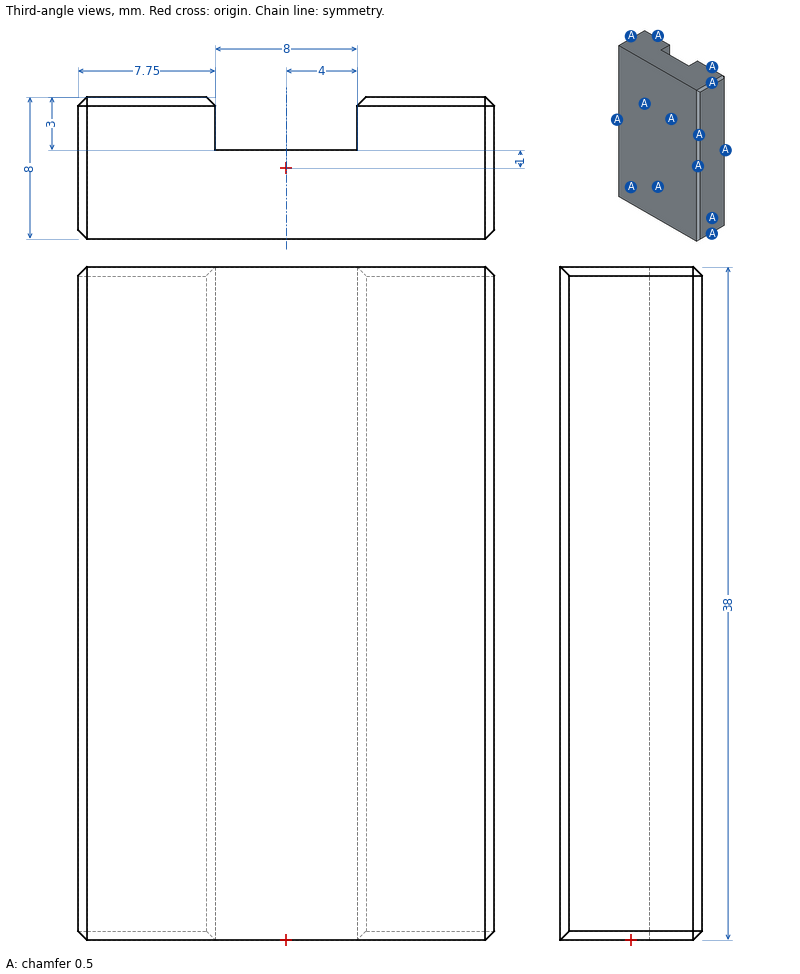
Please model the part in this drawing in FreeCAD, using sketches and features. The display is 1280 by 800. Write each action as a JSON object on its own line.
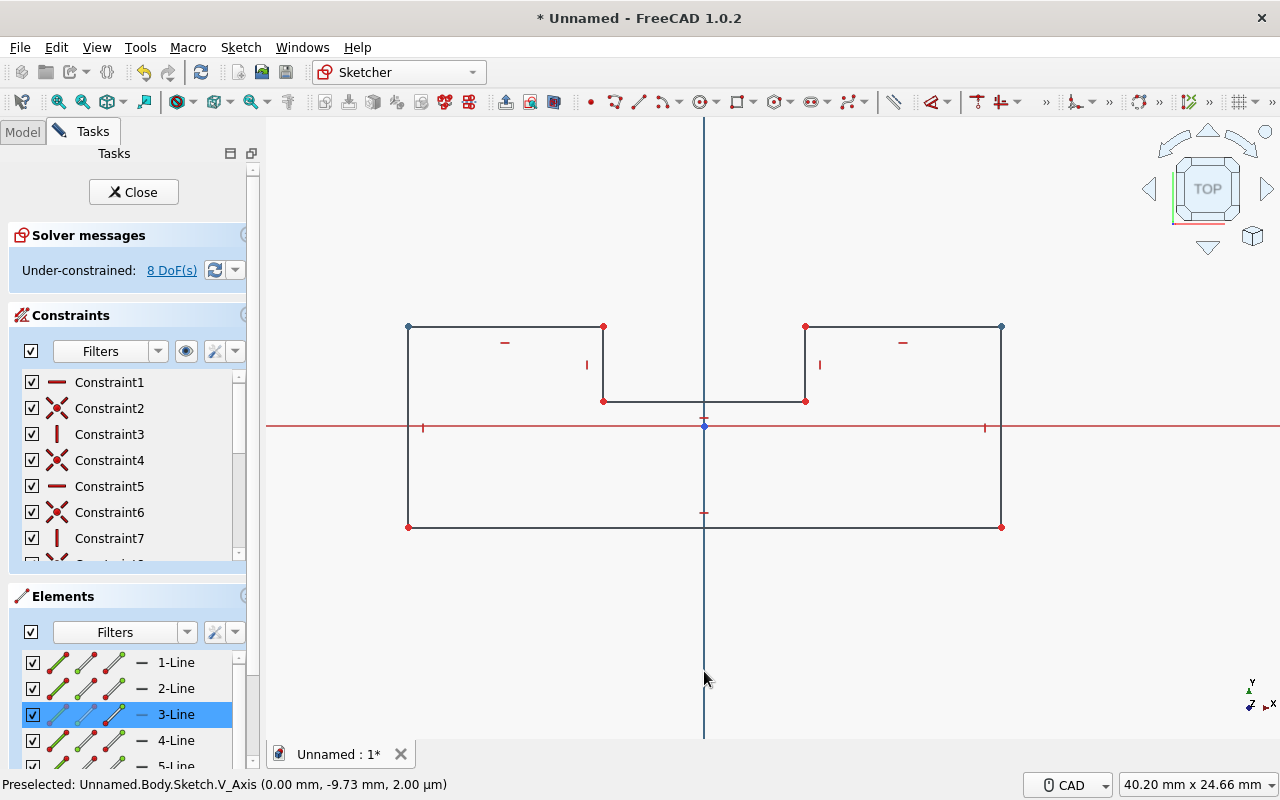
{"action": "key", "text": "s"}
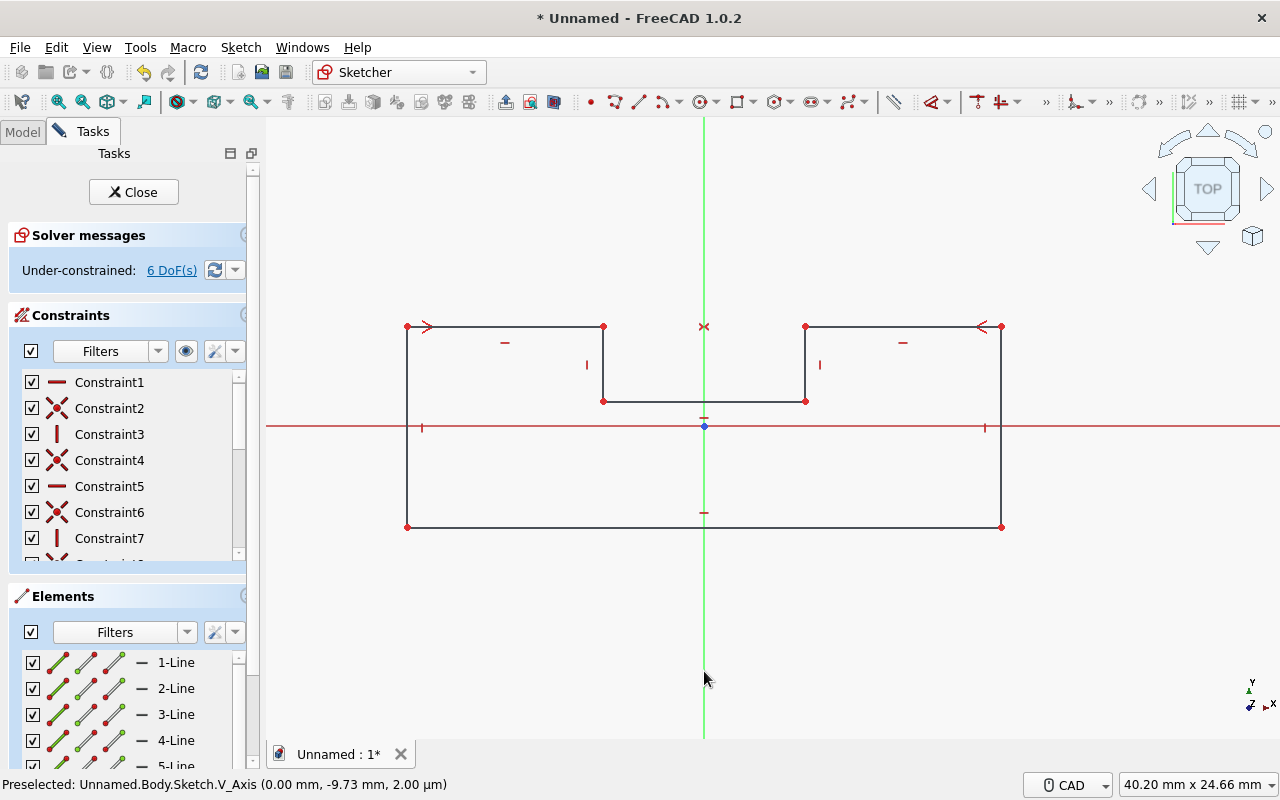
{"action": "left_click", "coordinate": [744, 402]}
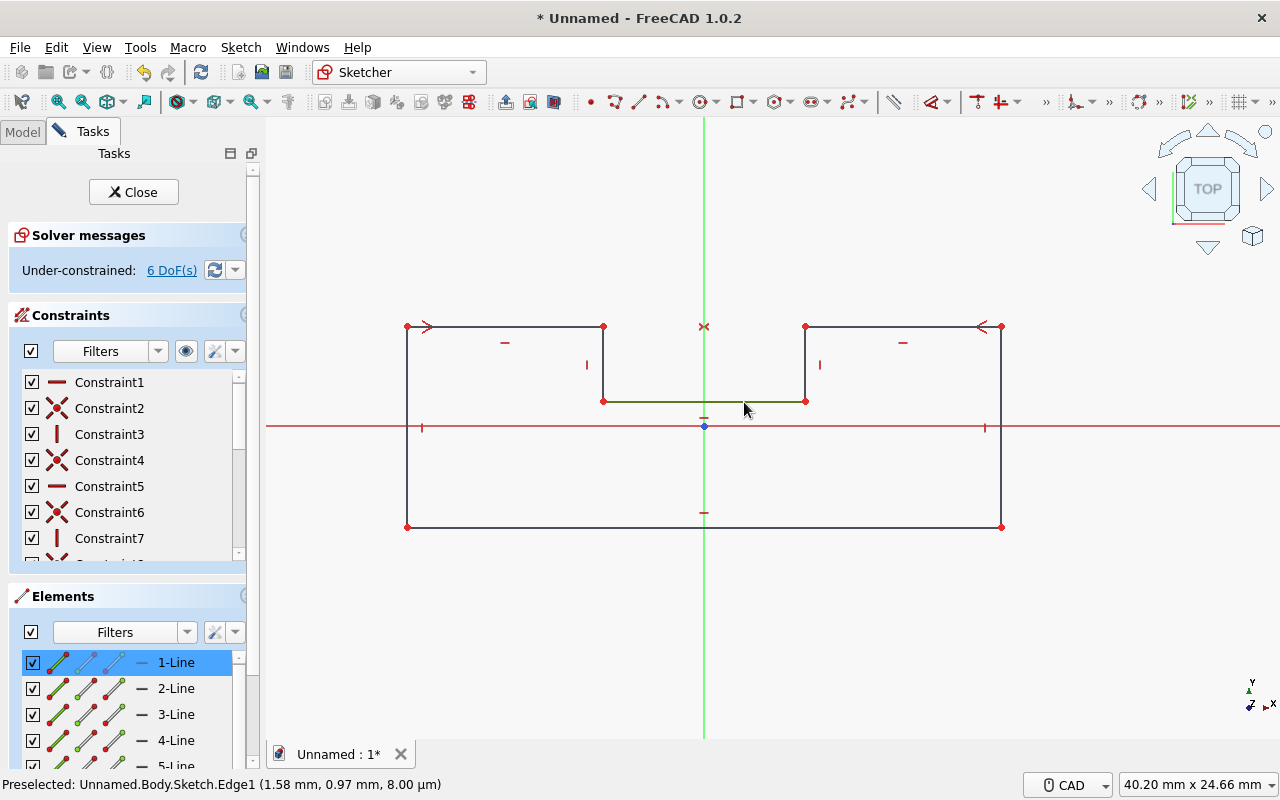
{"action": "left_click", "coordinate": [950, 102]}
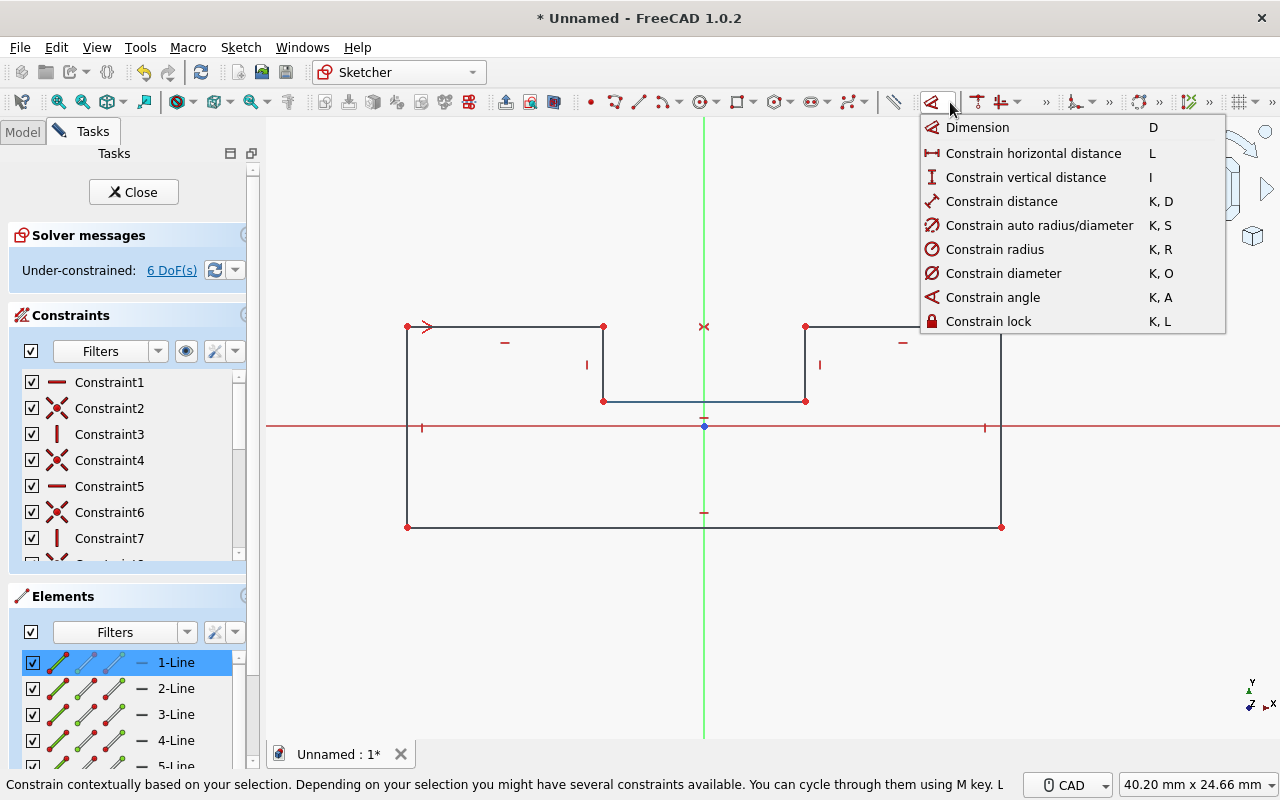
{"action": "left_click", "coordinate": [1073, 153]}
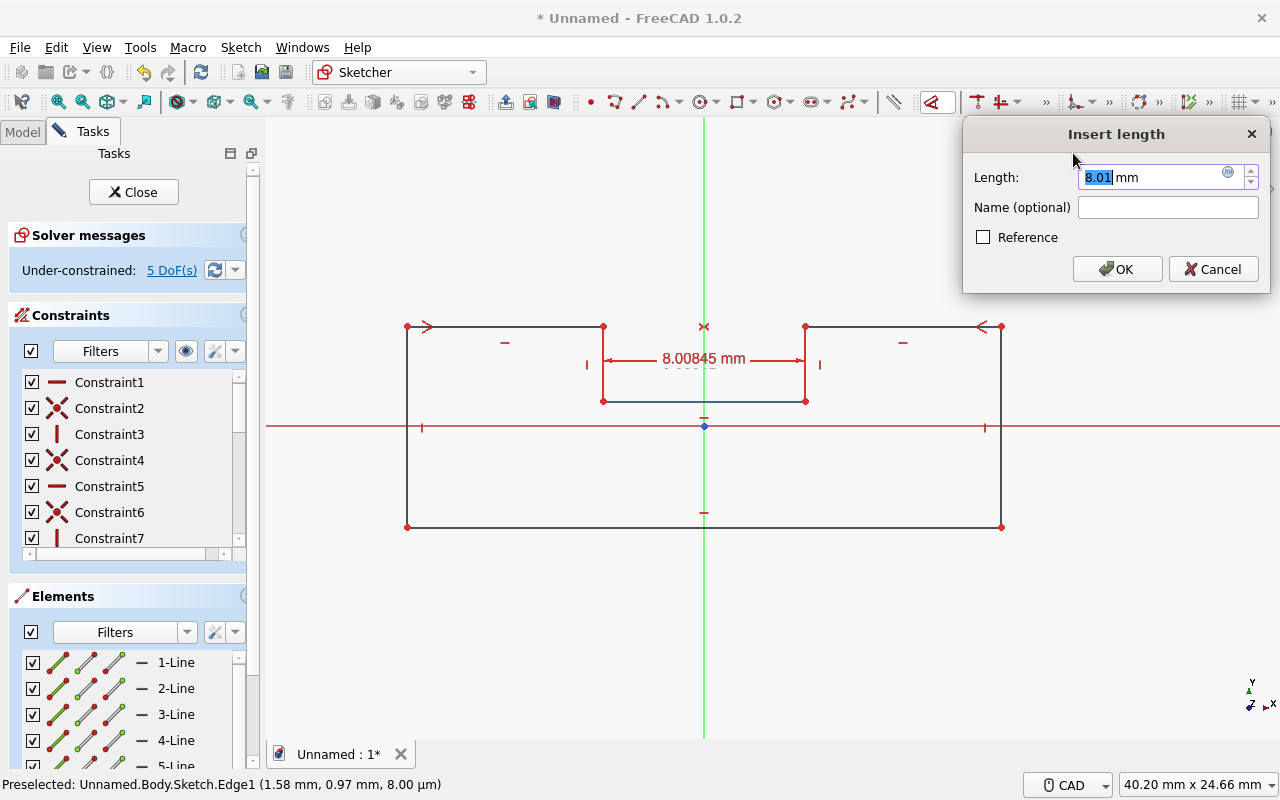
{"action": "type", "text": "8"}
{"action": "key", "text": "Return"}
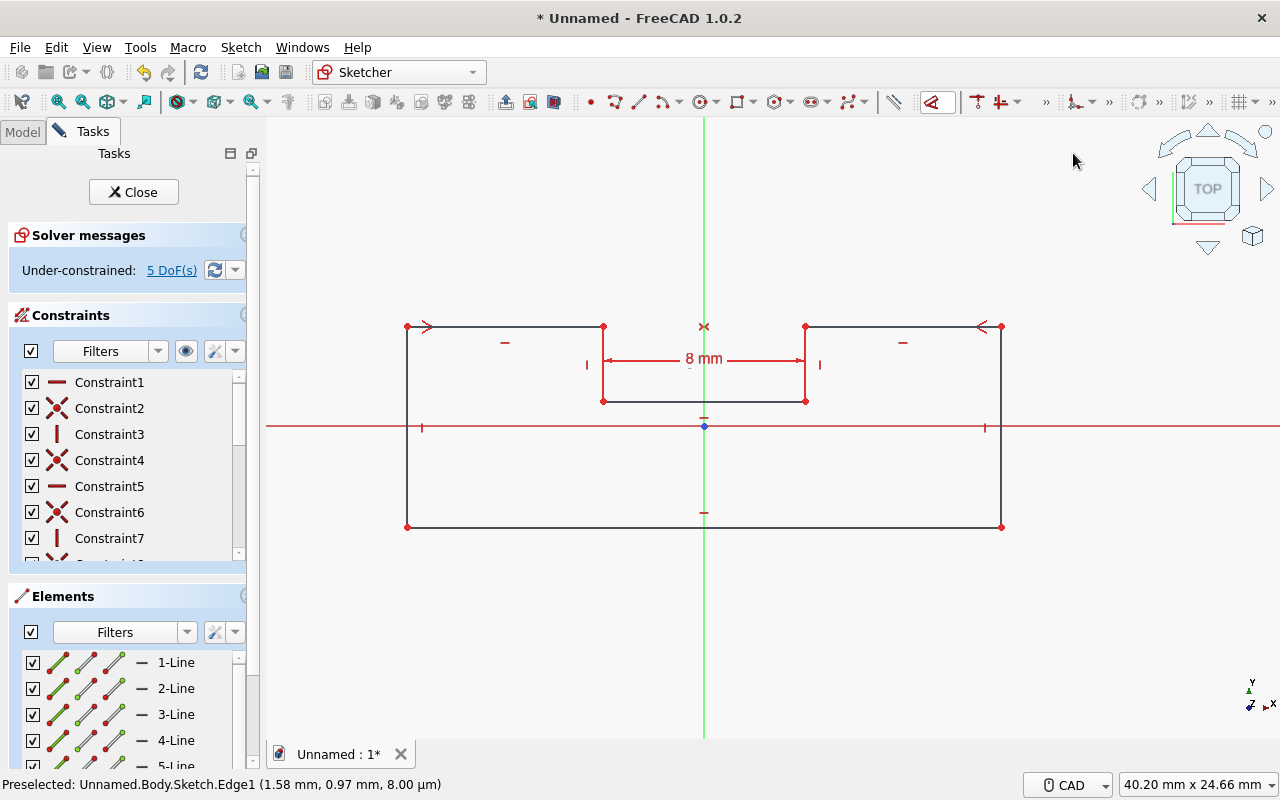
{"action": "left_click", "coordinate": [603, 380]}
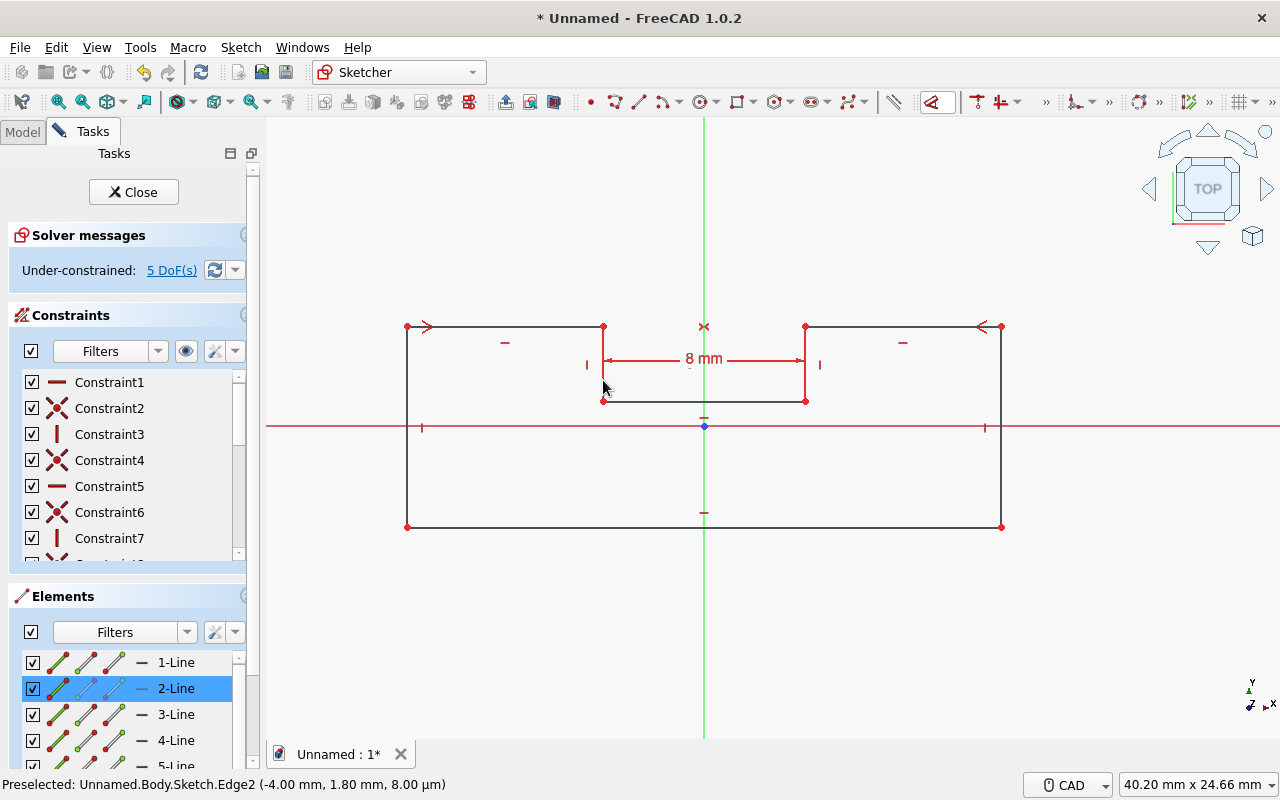
{"action": "key", "text": "i"}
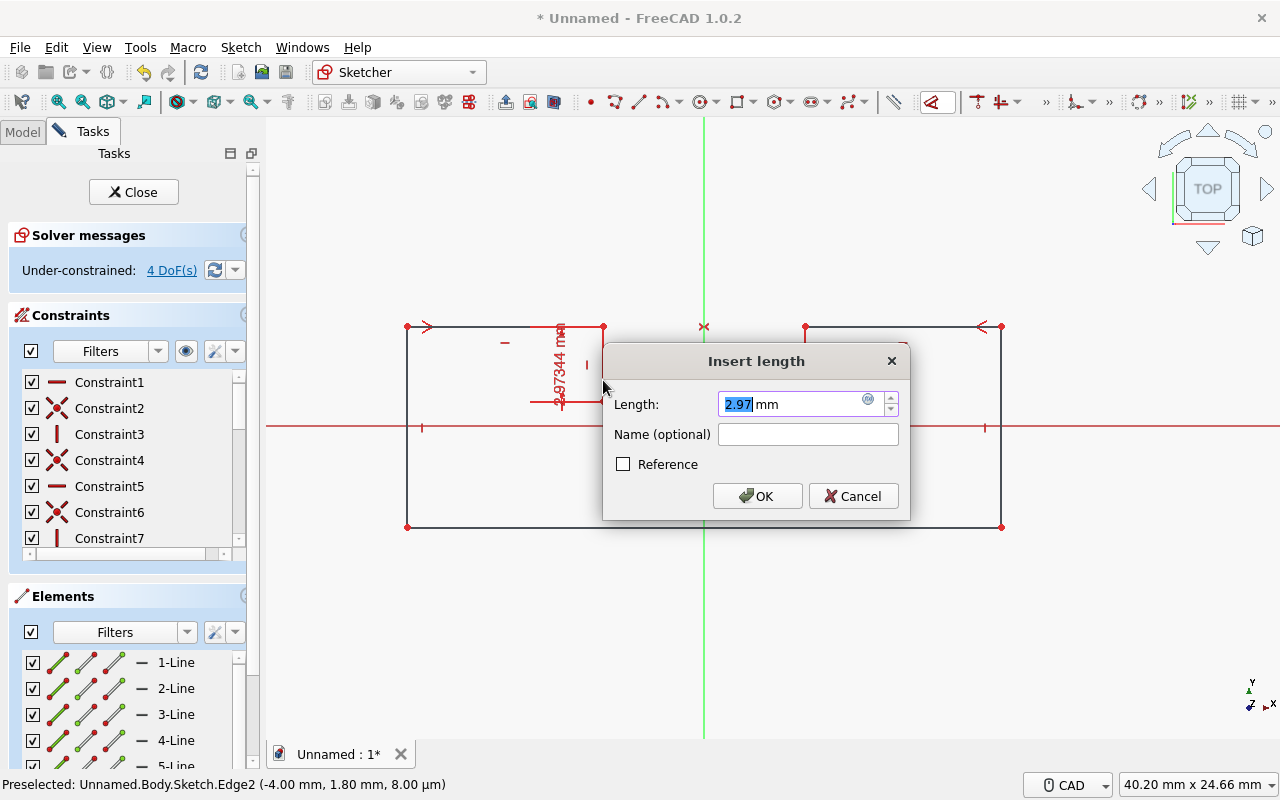
{"action": "type", "text": "3"}
{"action": "key", "text": "Return"}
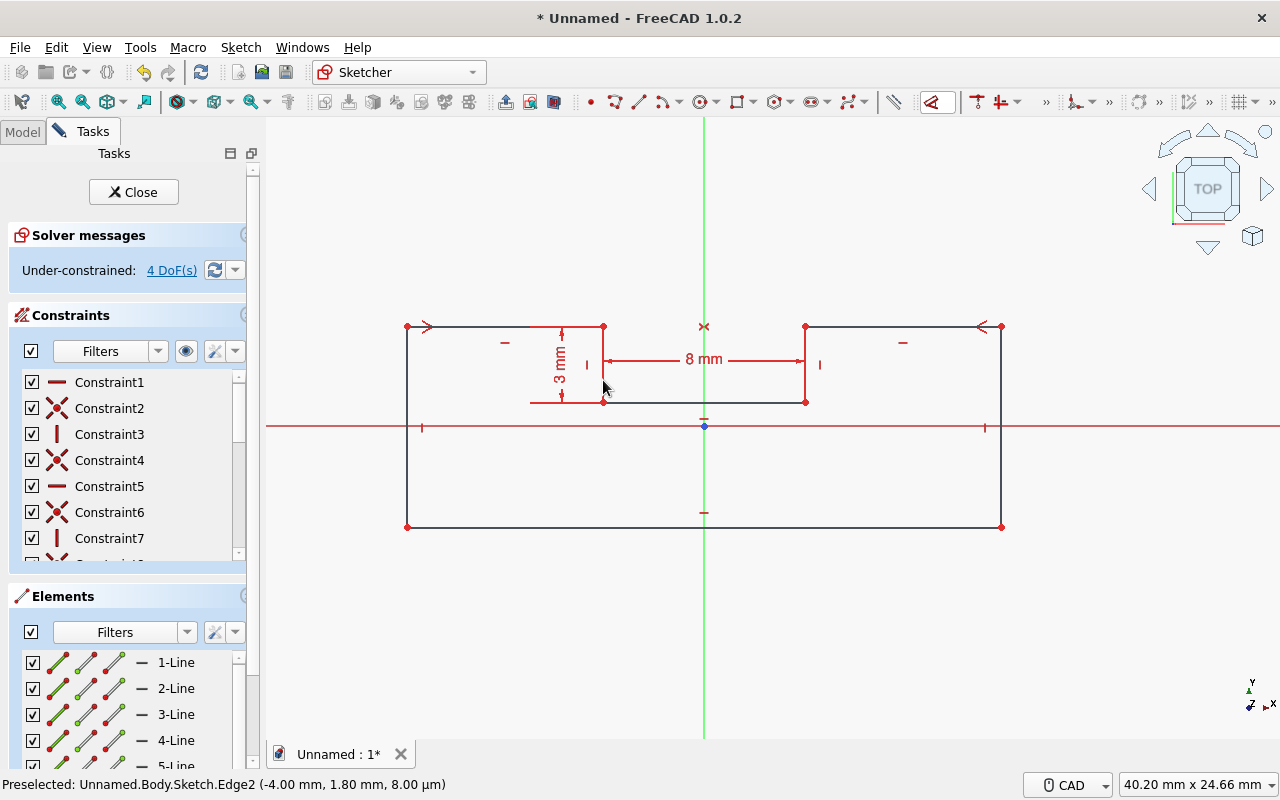
{"action": "left_click", "coordinate": [407, 387]}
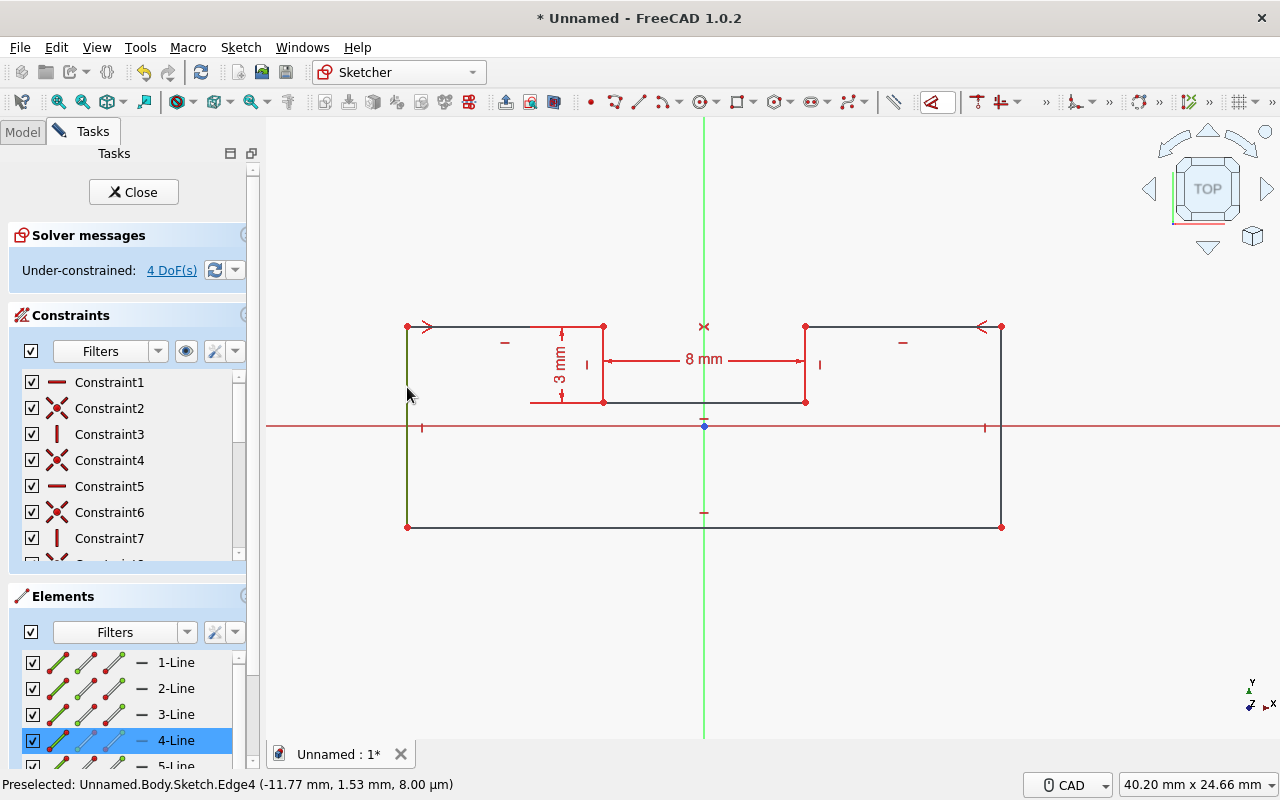
{"action": "key", "text": "i"}